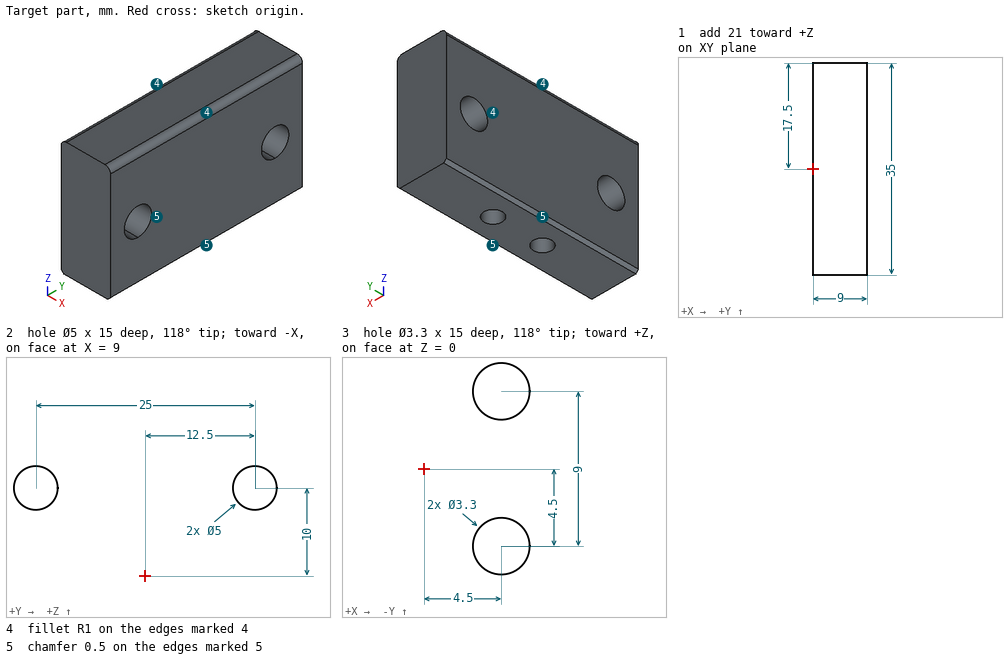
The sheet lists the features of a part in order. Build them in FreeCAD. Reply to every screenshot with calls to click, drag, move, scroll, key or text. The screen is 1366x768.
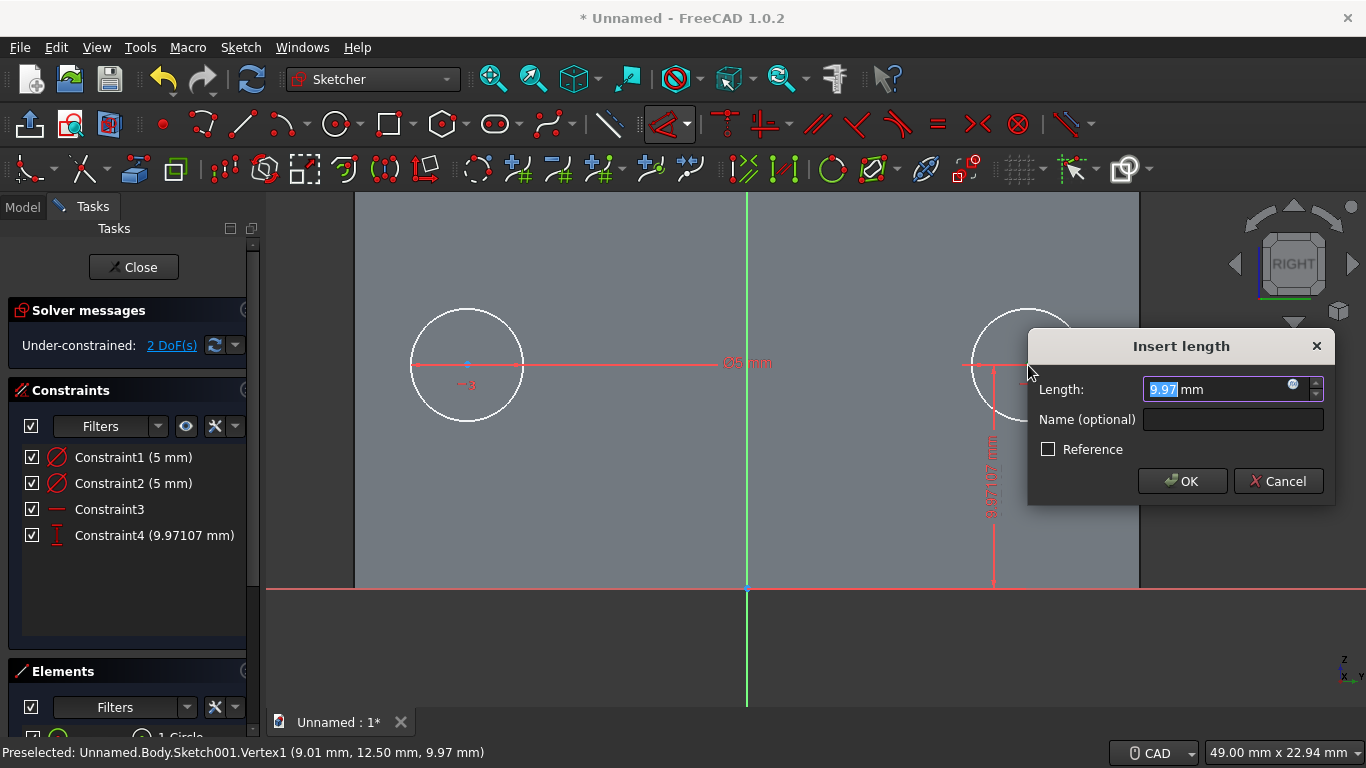
text(10)
key(Return)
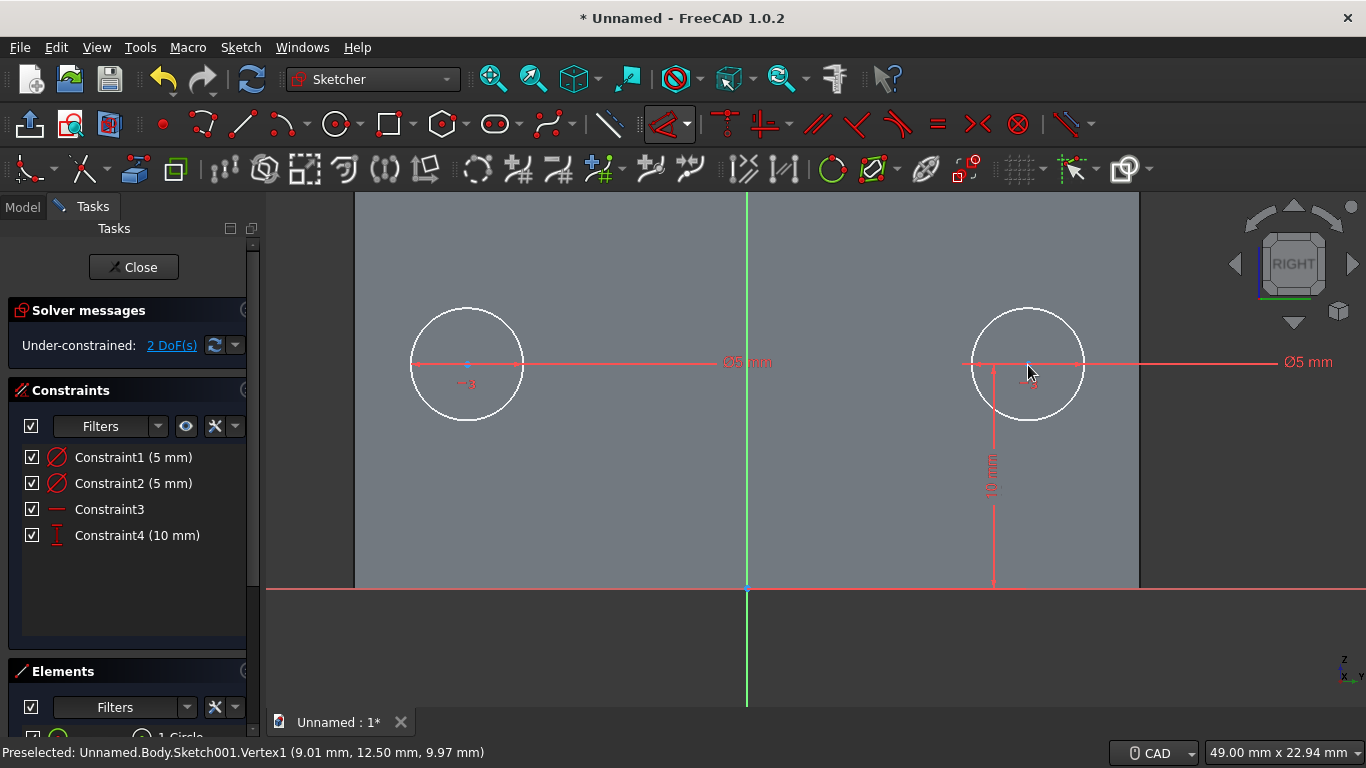
click(1028, 364)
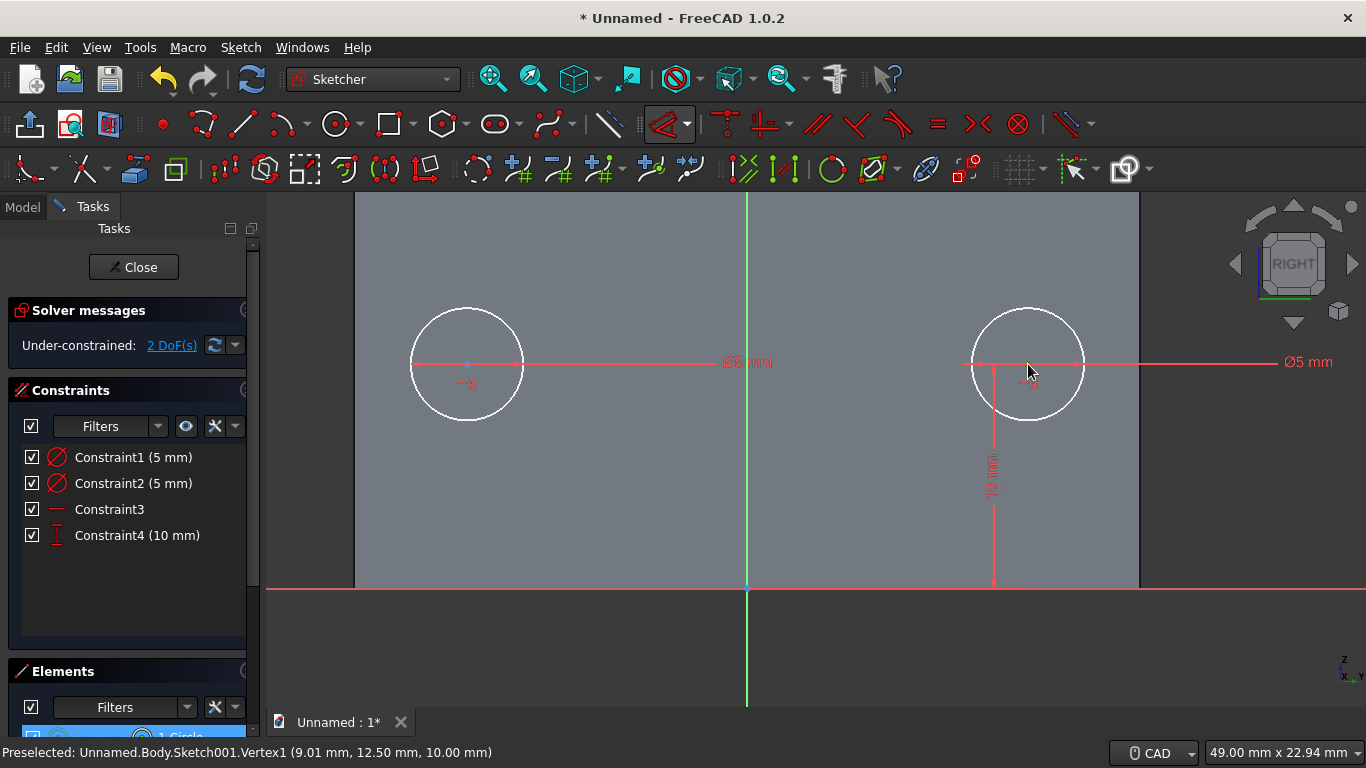
click(467, 364)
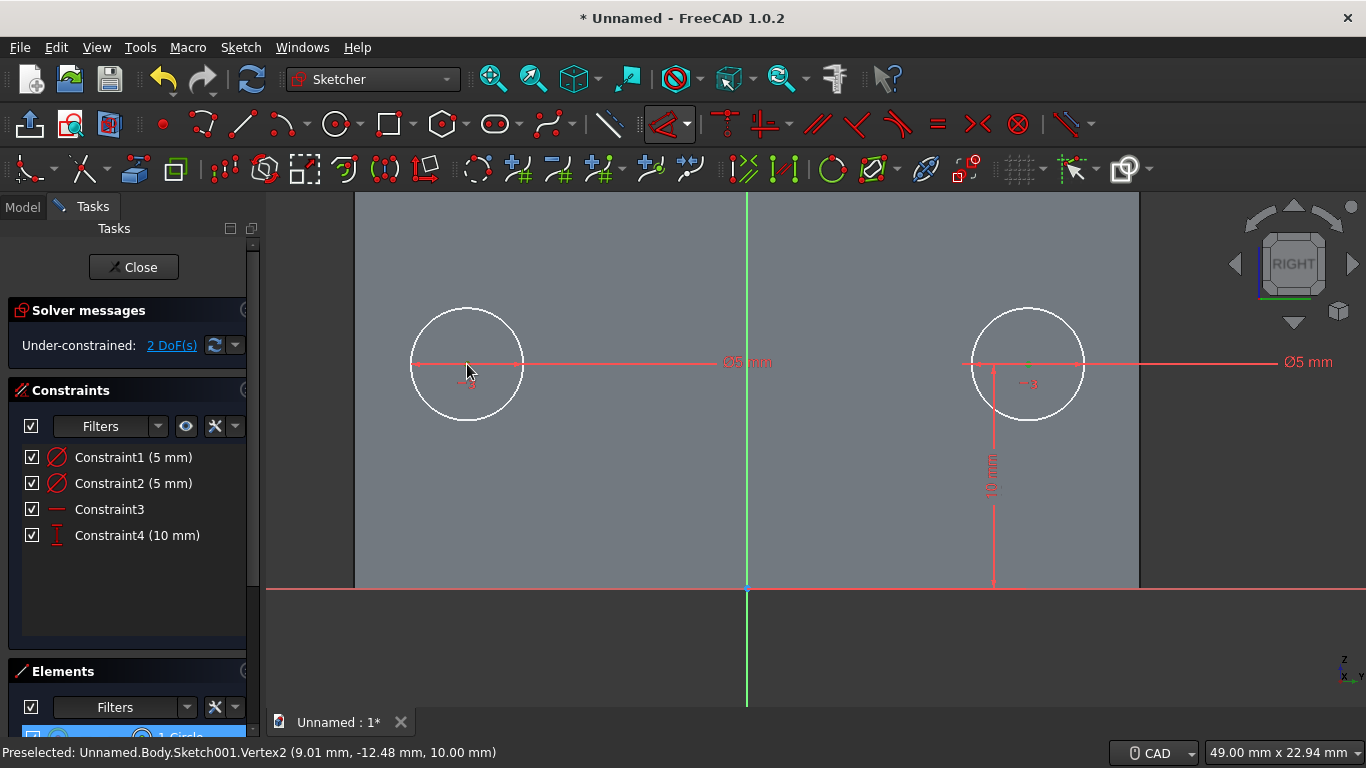
key(l)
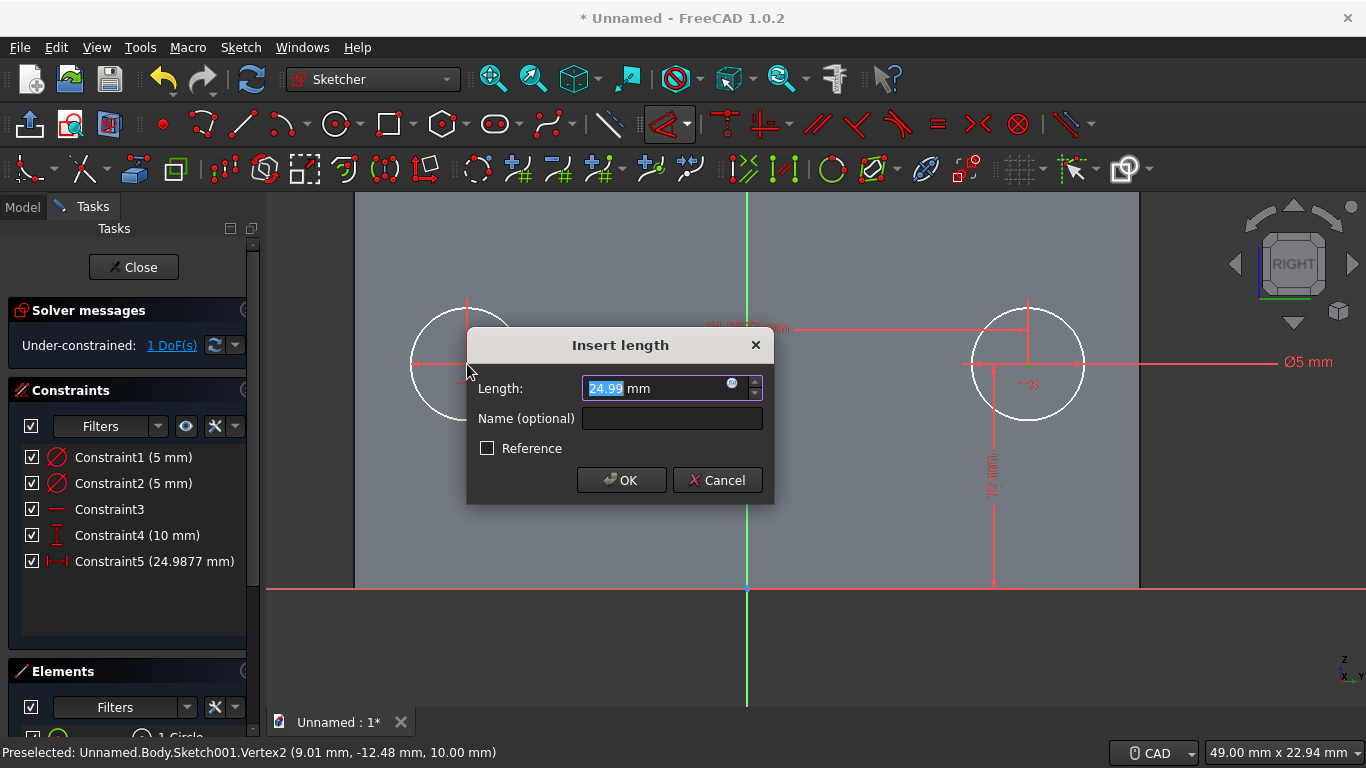
text(25)
key(Return)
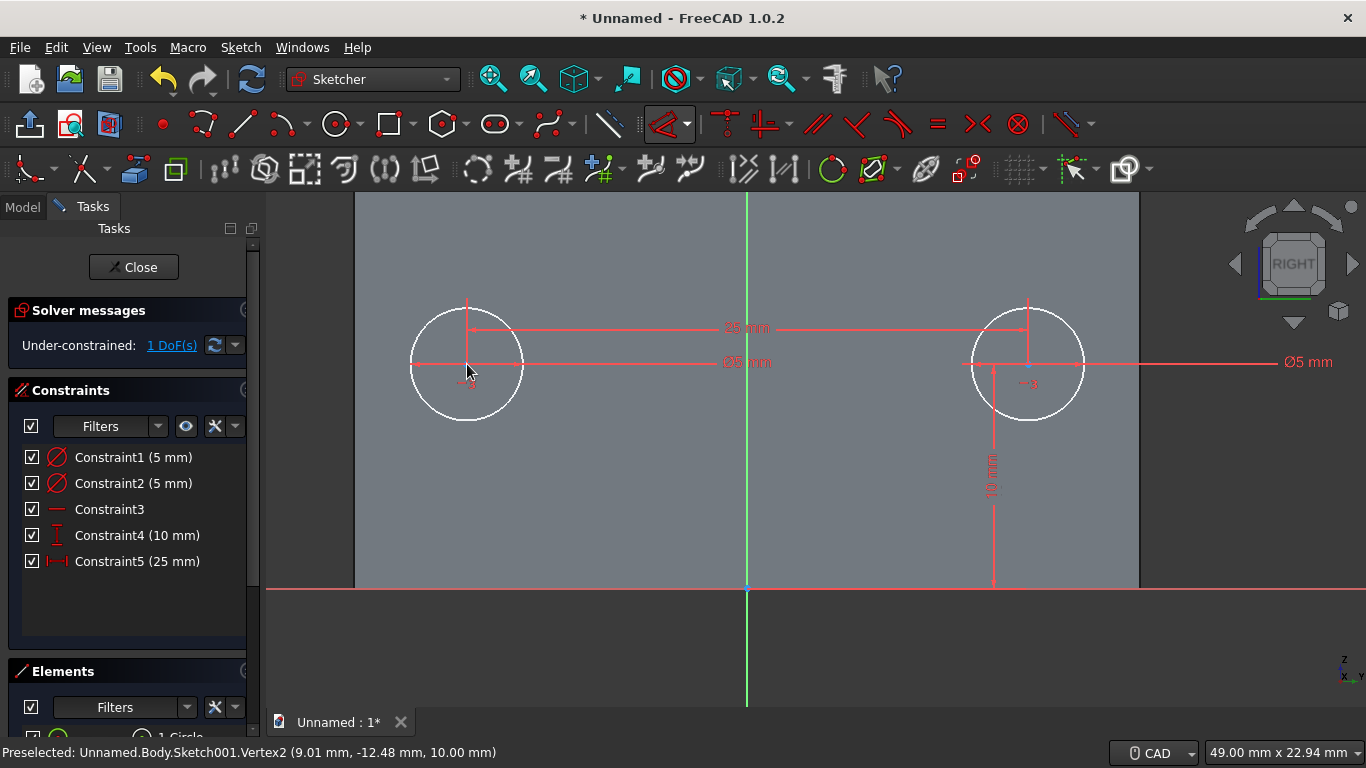
click(1028, 364)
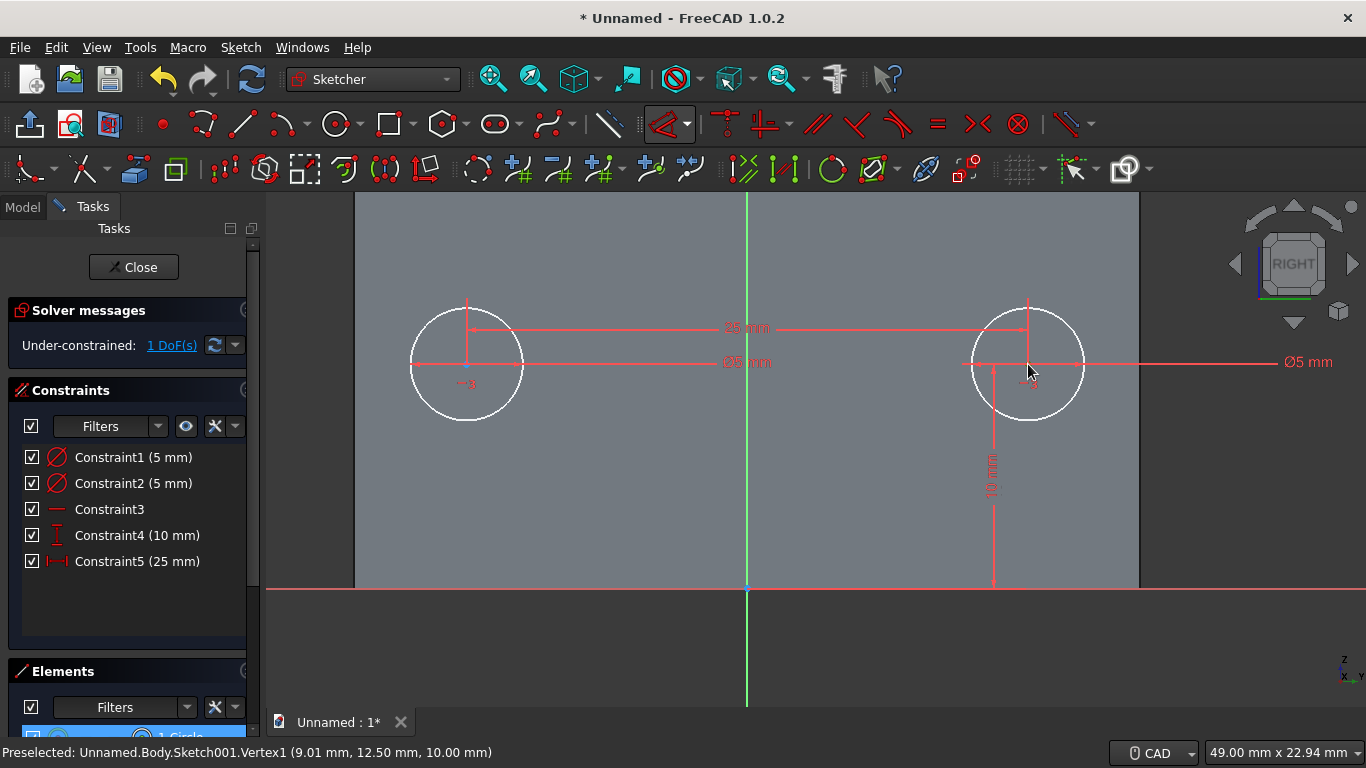
key(l)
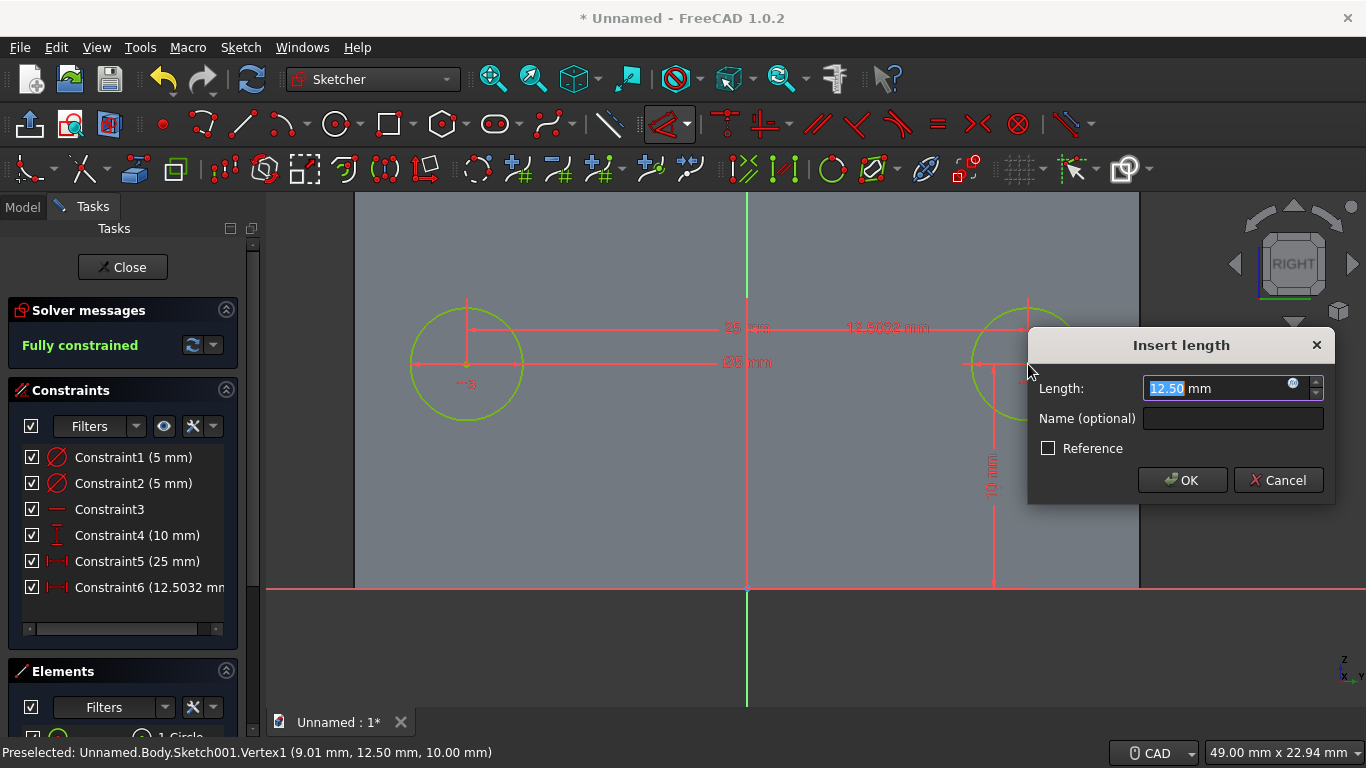
text(12.5)
key(Return)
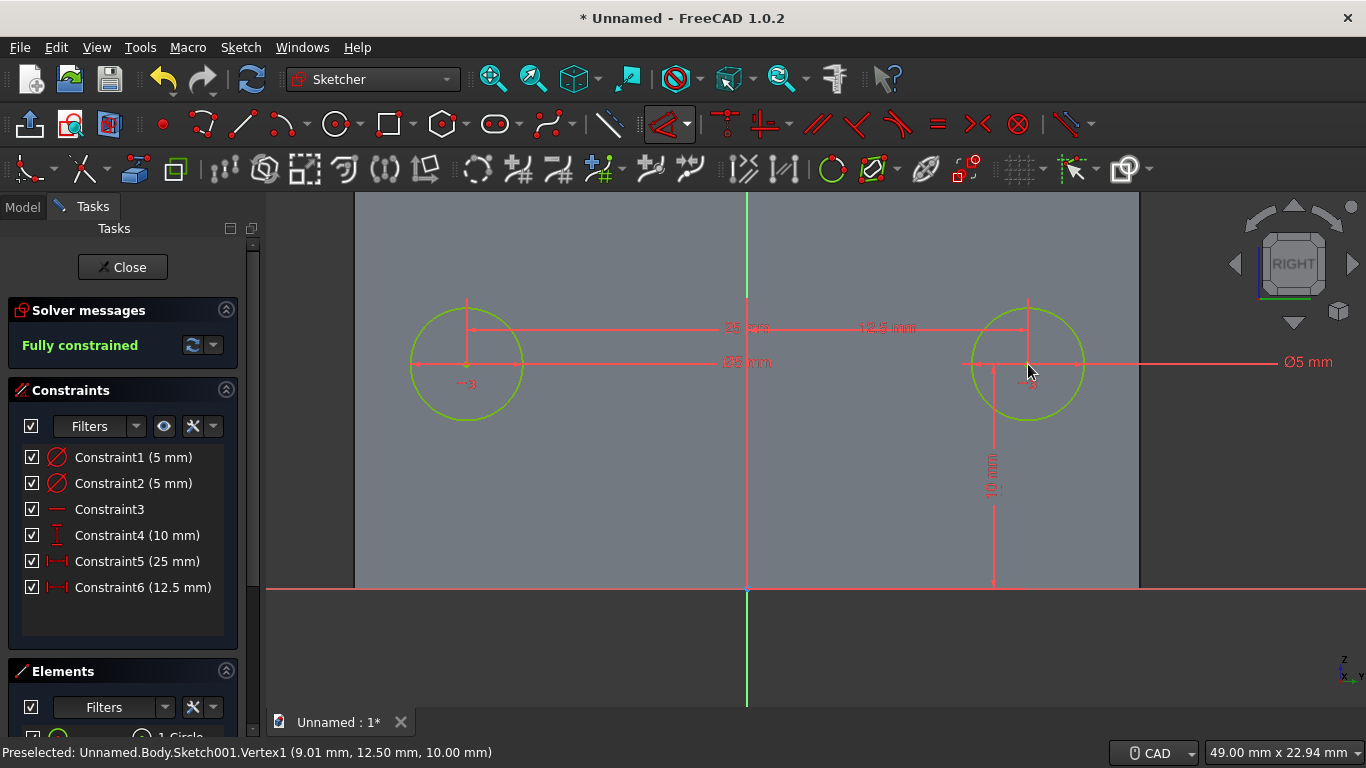
click(123, 267)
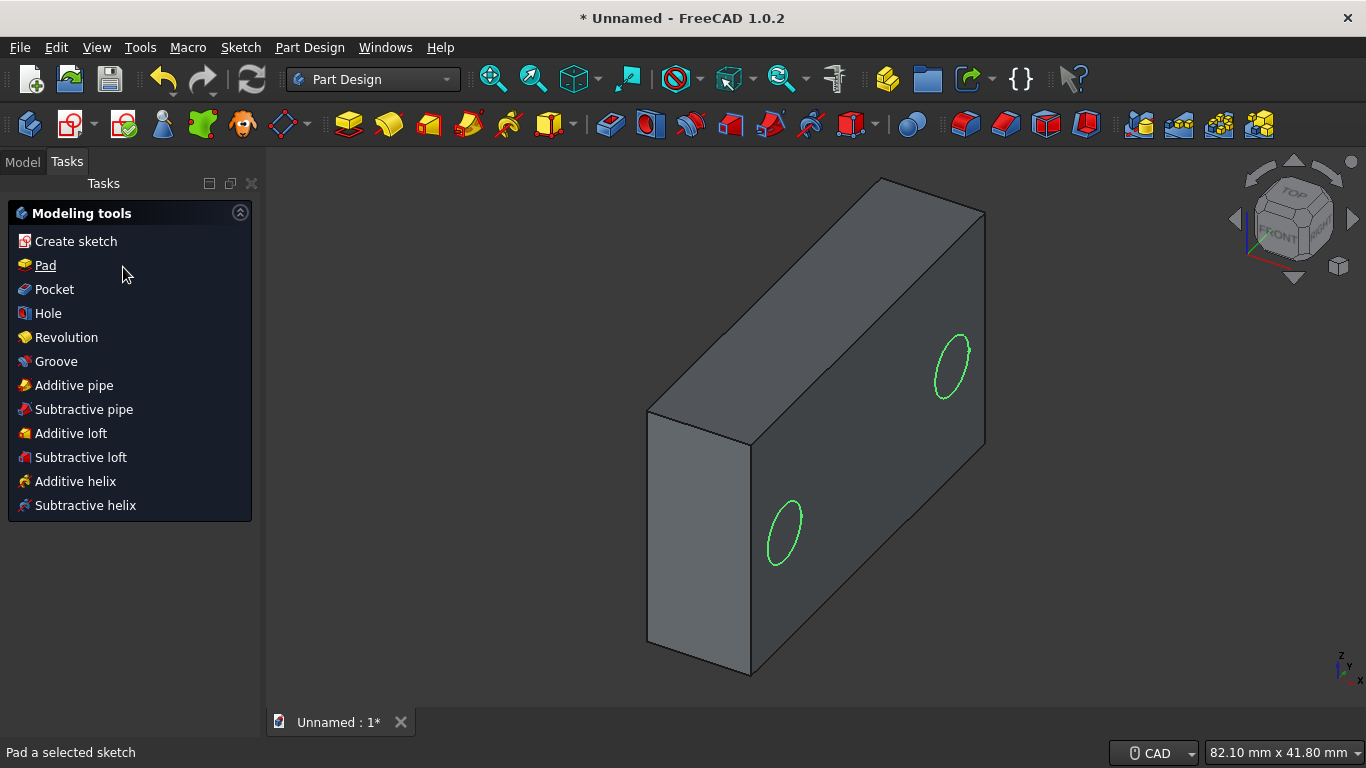
click(652, 124)